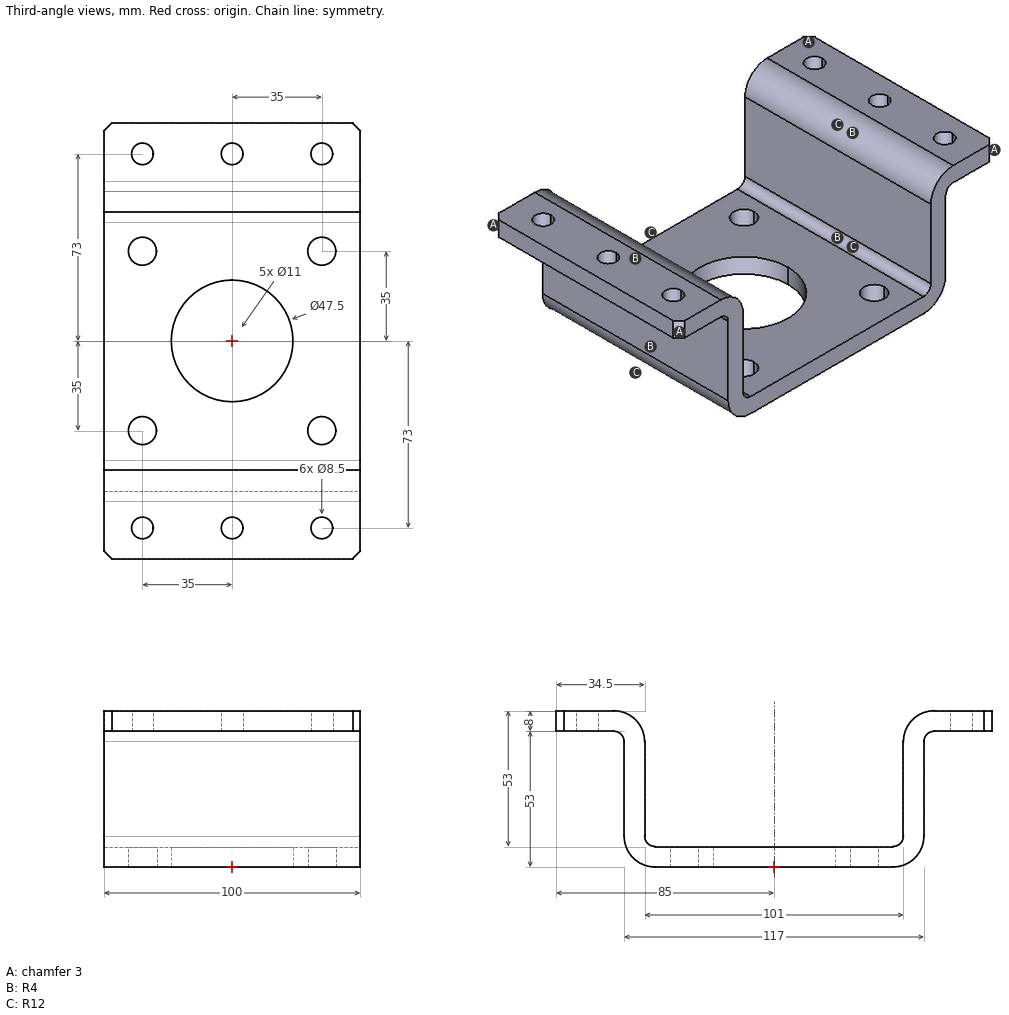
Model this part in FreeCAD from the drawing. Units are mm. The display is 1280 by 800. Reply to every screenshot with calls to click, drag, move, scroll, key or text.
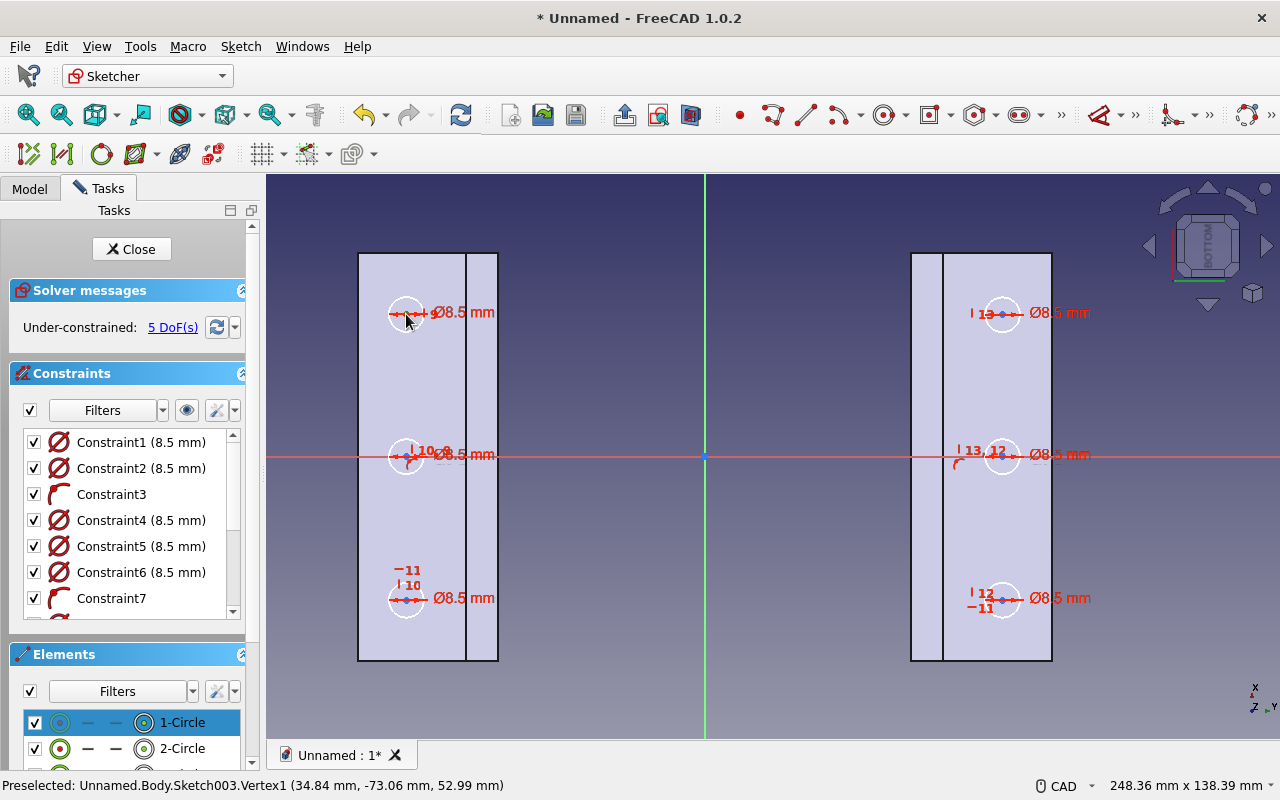
click(1003, 315)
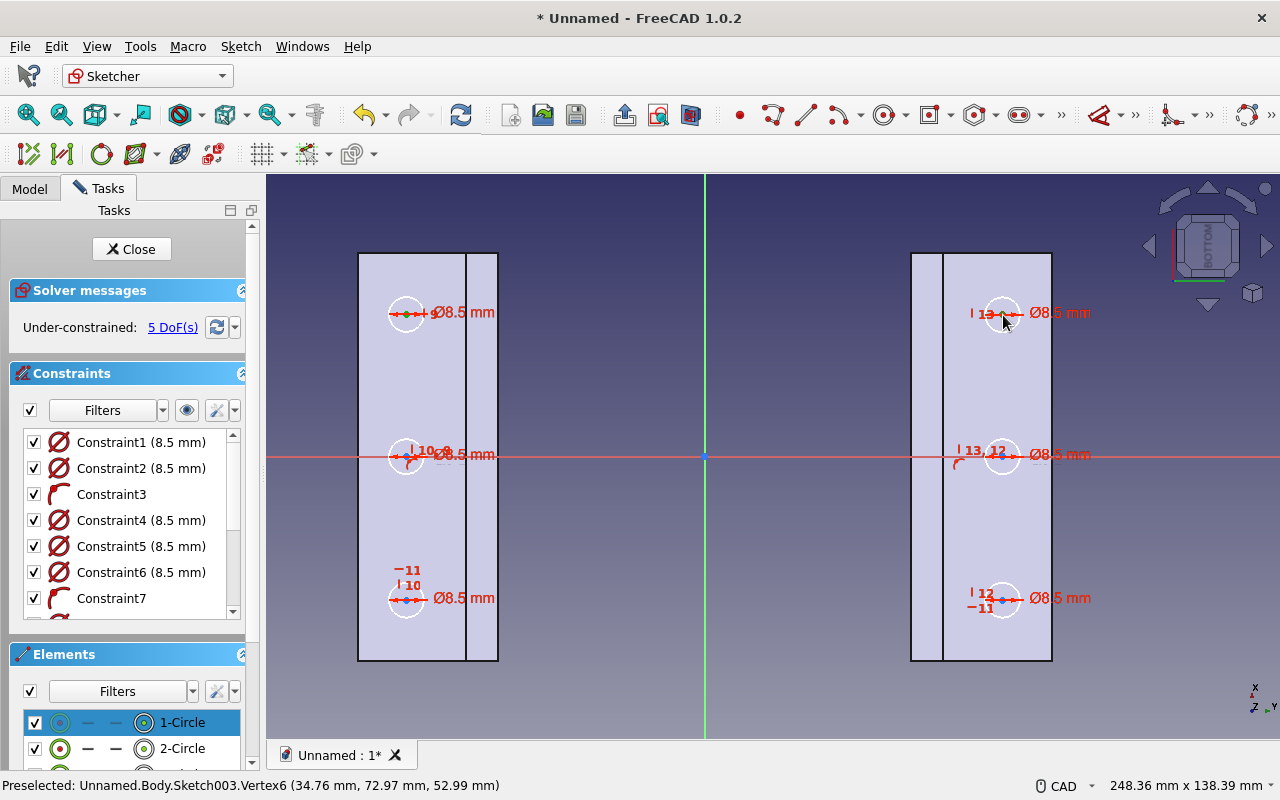
key(h)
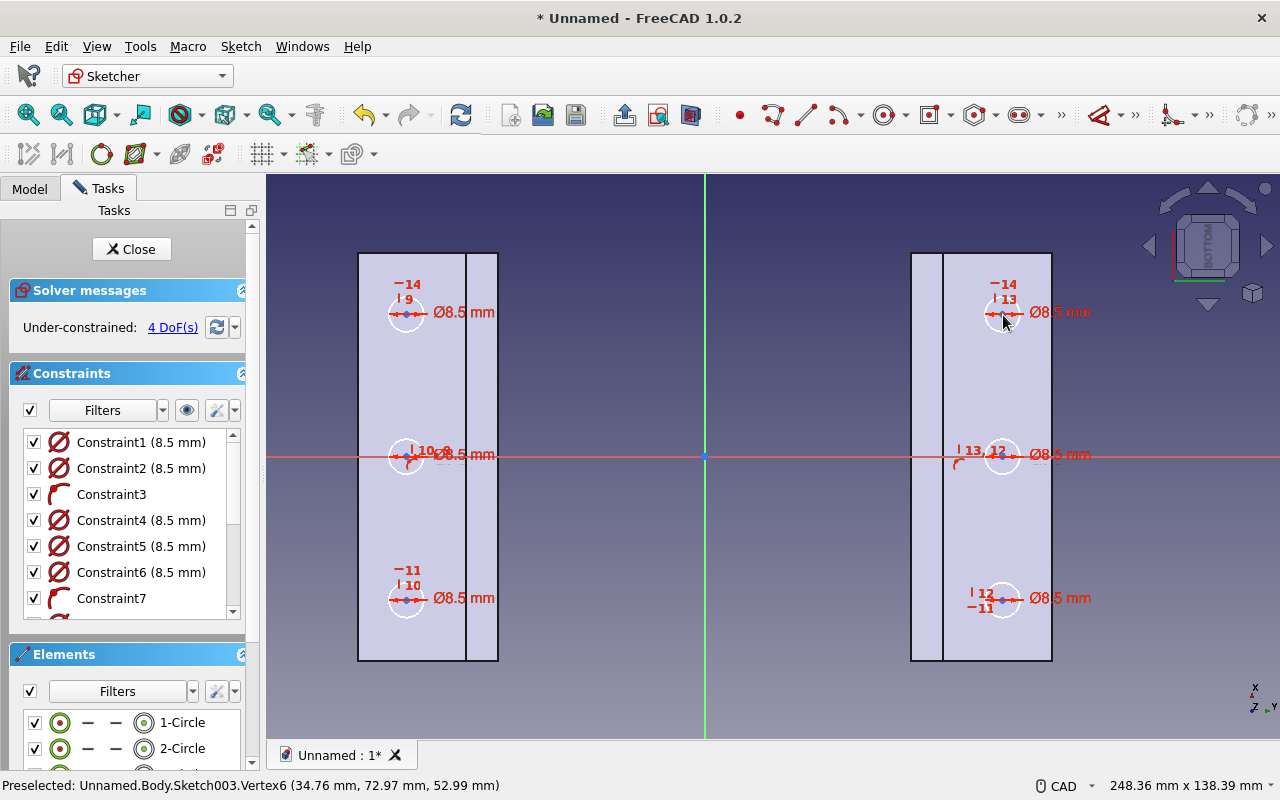
key(d)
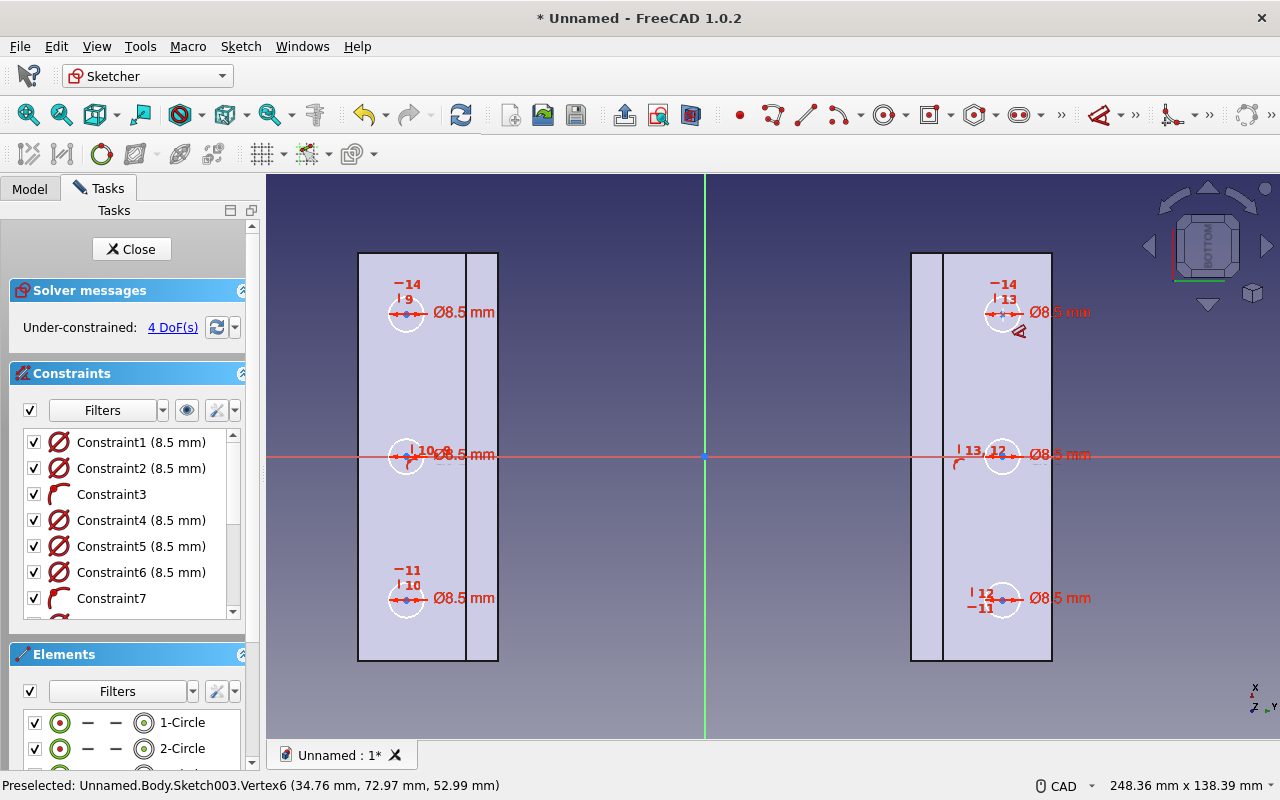
click(406, 314)
click(556, 280)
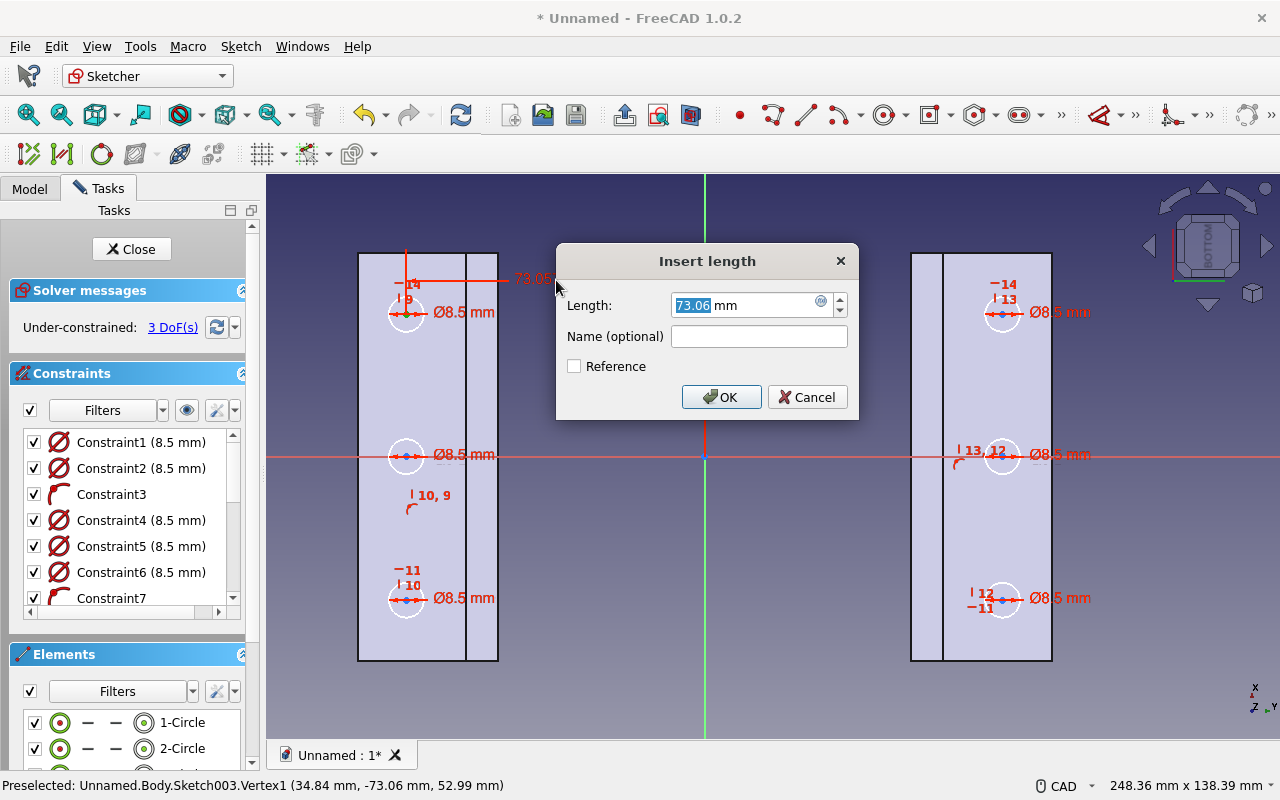
text(73)
key(Return)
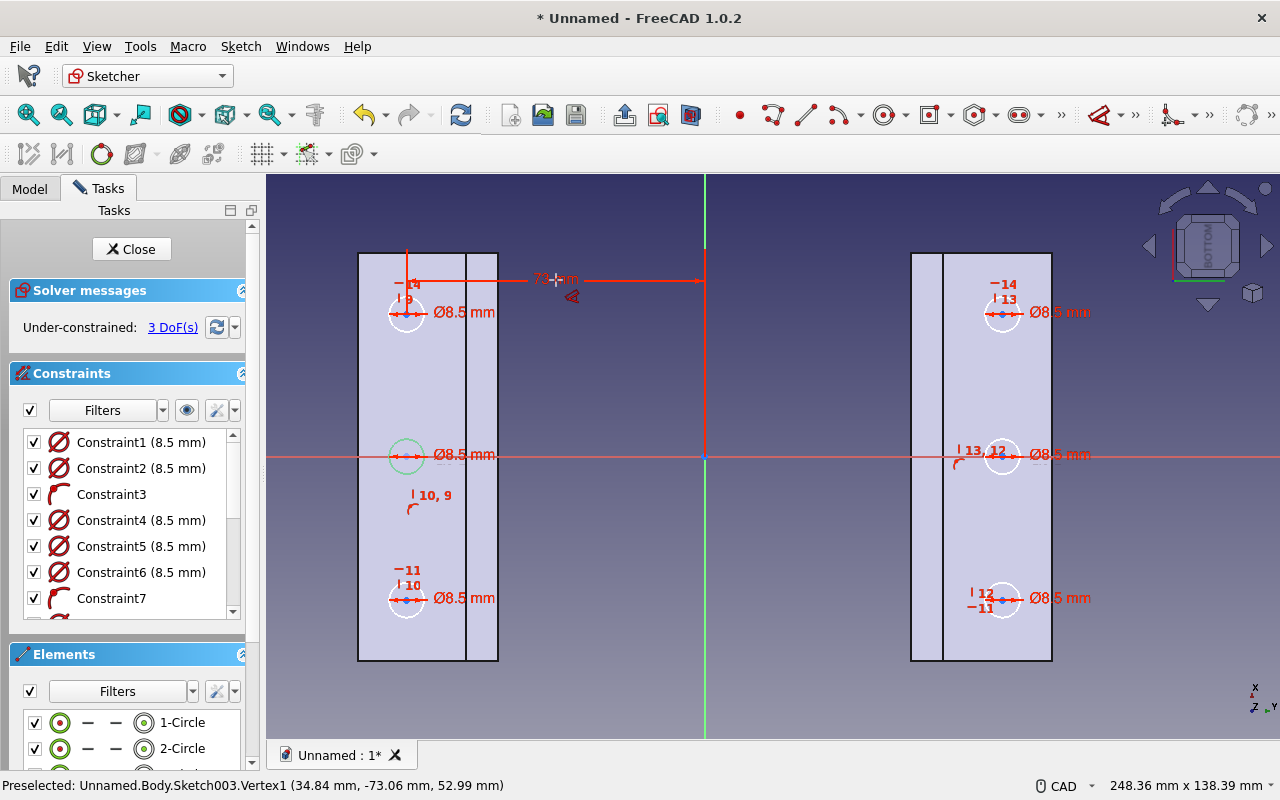
click(407, 314)
click(373, 386)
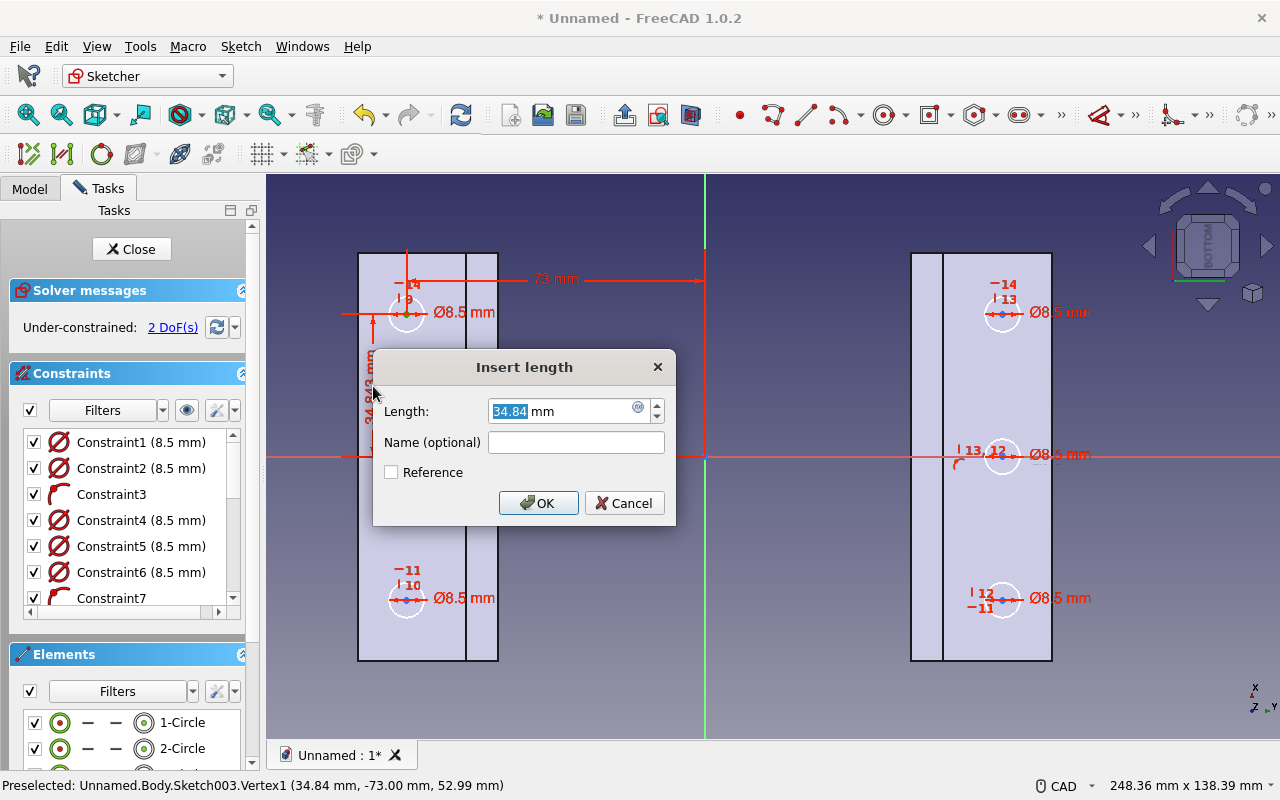
text(35)
key(Return)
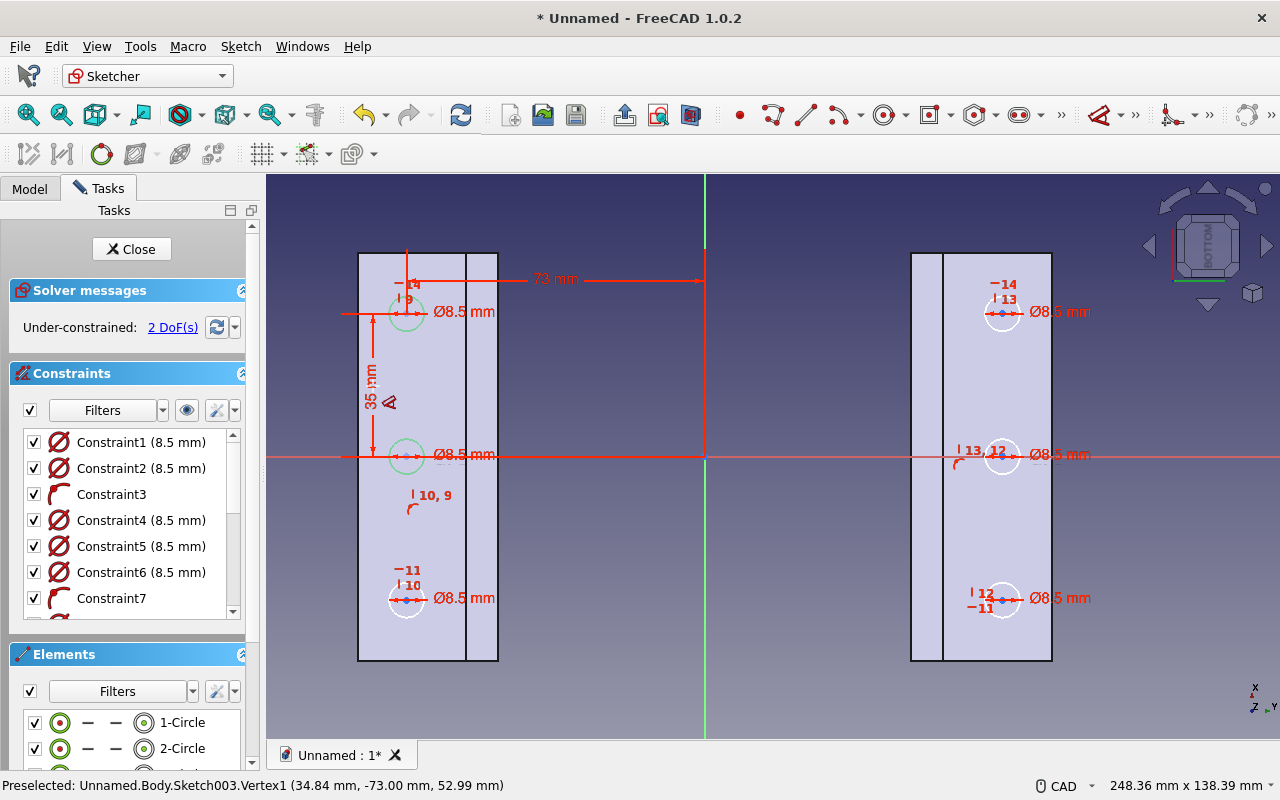
click(407, 600)
click(373, 528)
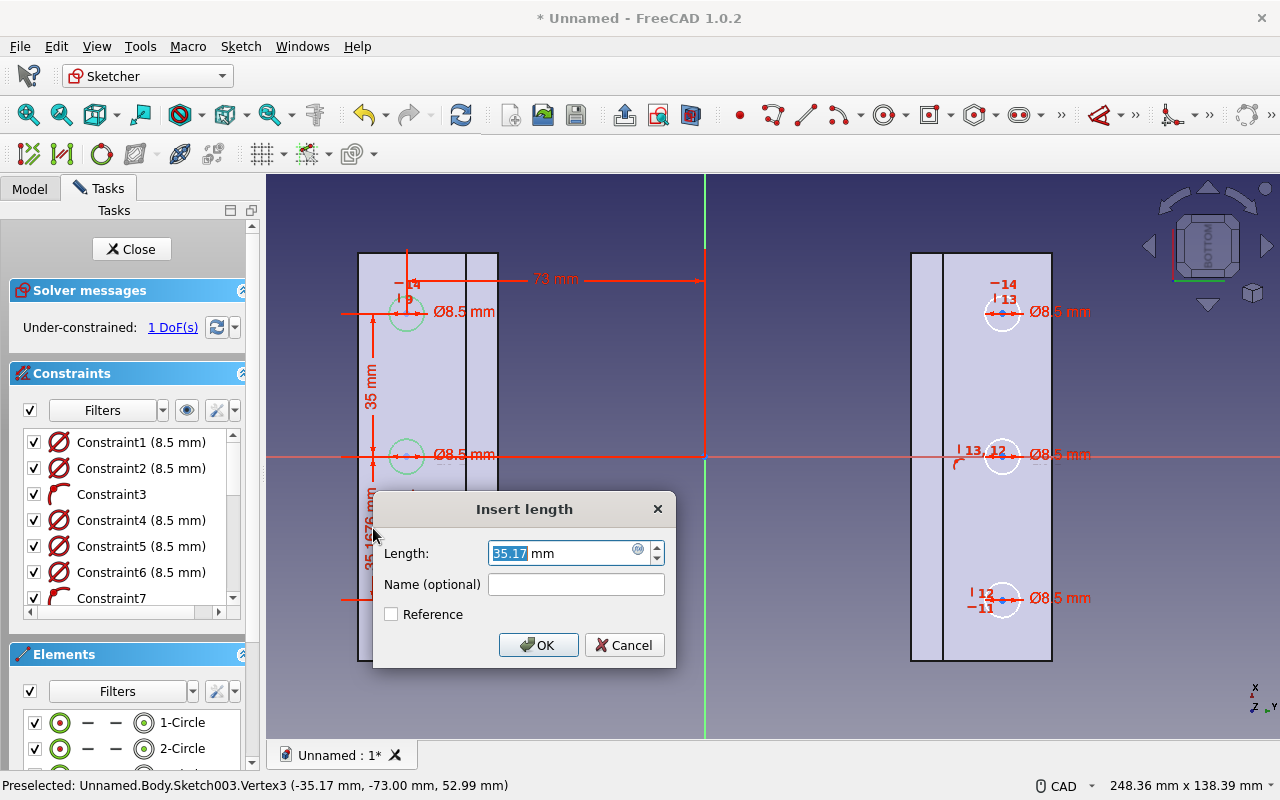
text(35)
key(Return)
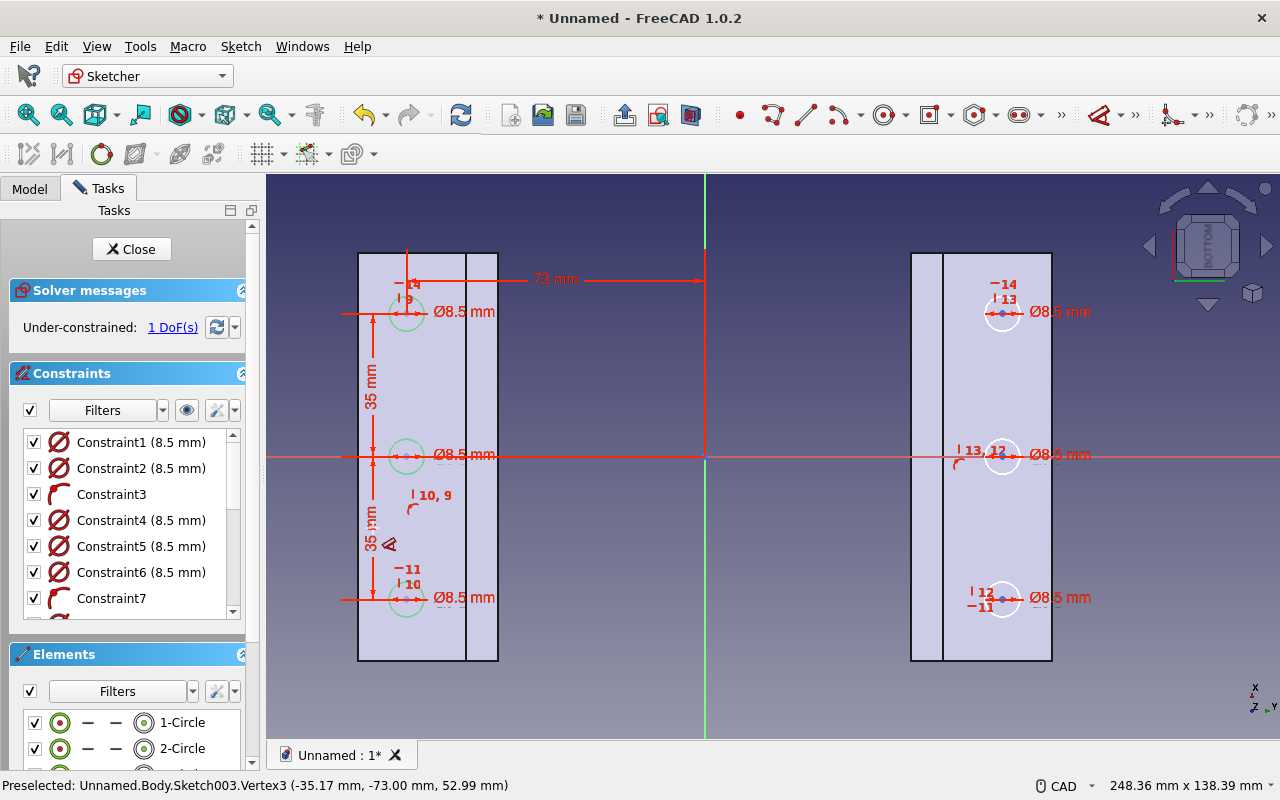
click(1003, 600)
click(854, 634)